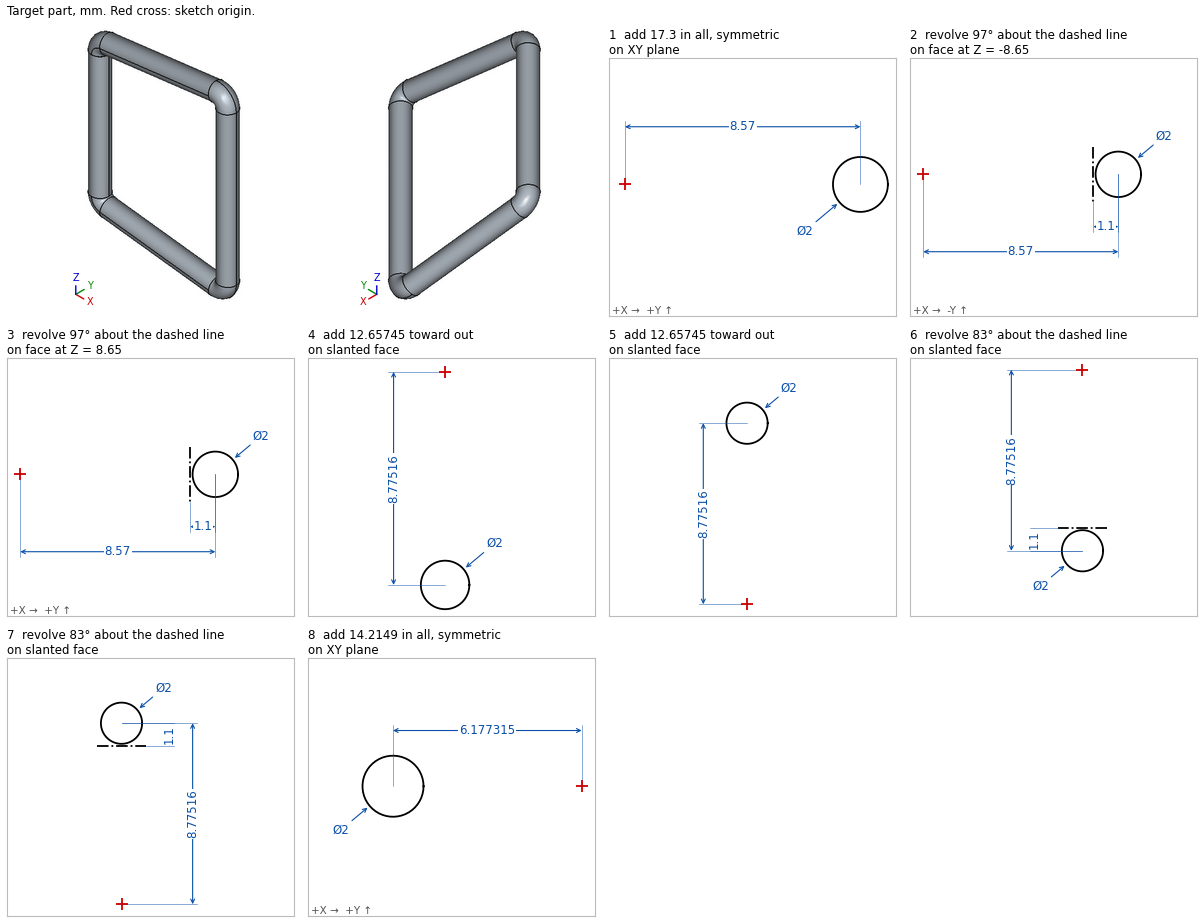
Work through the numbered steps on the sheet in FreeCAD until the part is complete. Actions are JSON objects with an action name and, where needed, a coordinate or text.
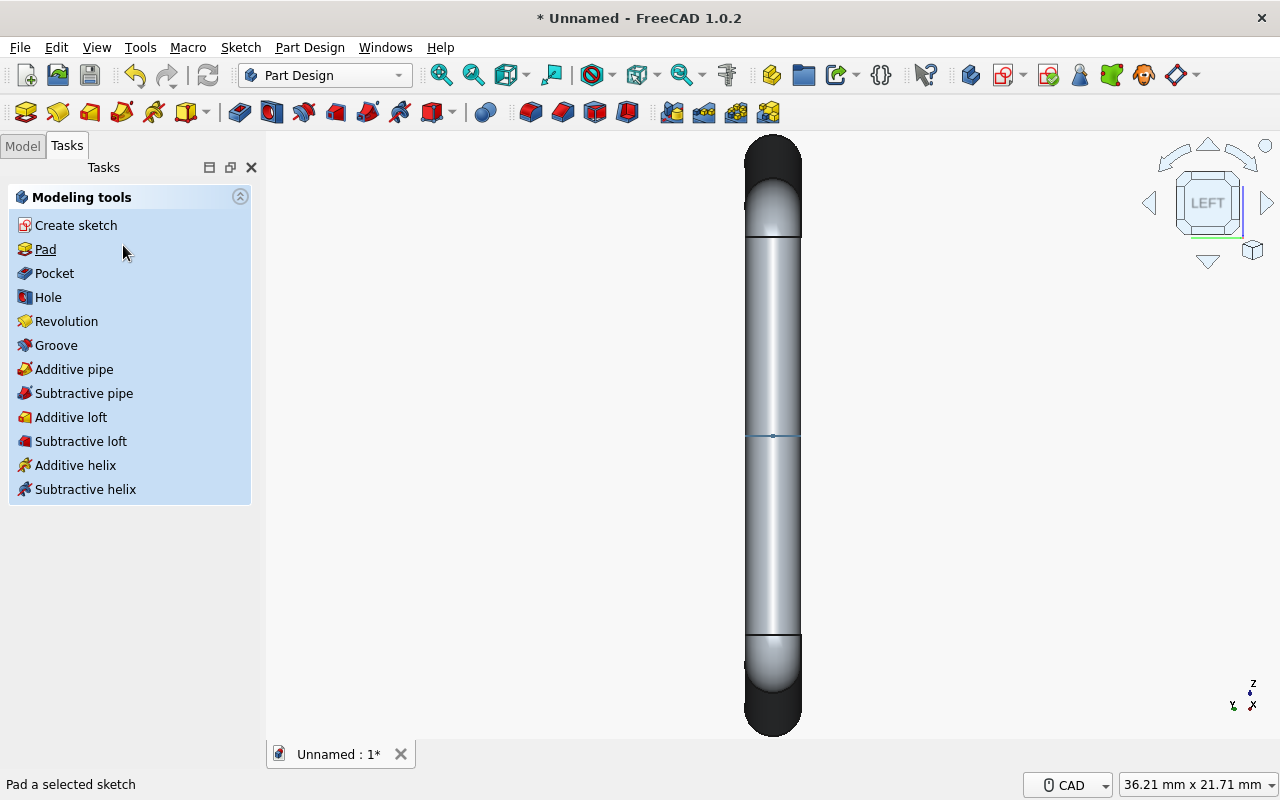
{"action": "left_click", "coordinate": [26, 112]}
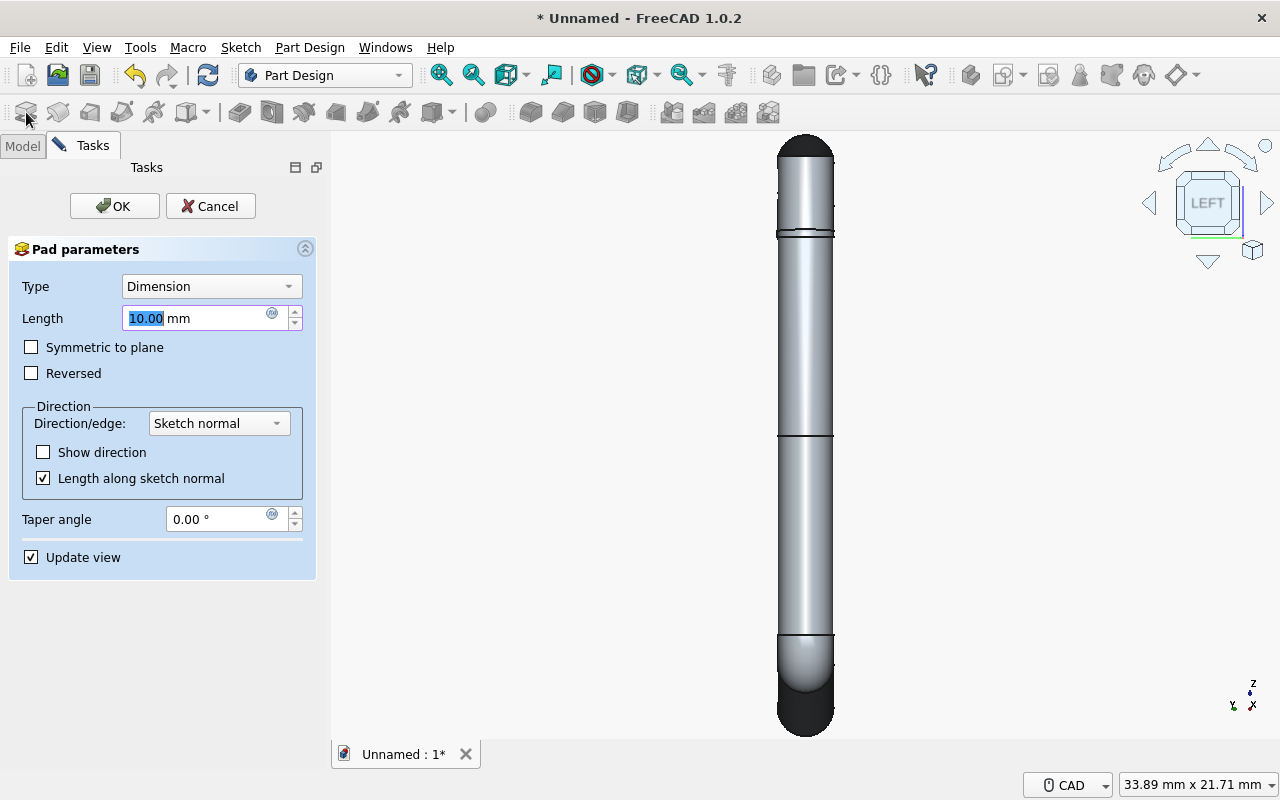
{"action": "type", "text": "14.2149"}
{"action": "key", "text": "Tab"}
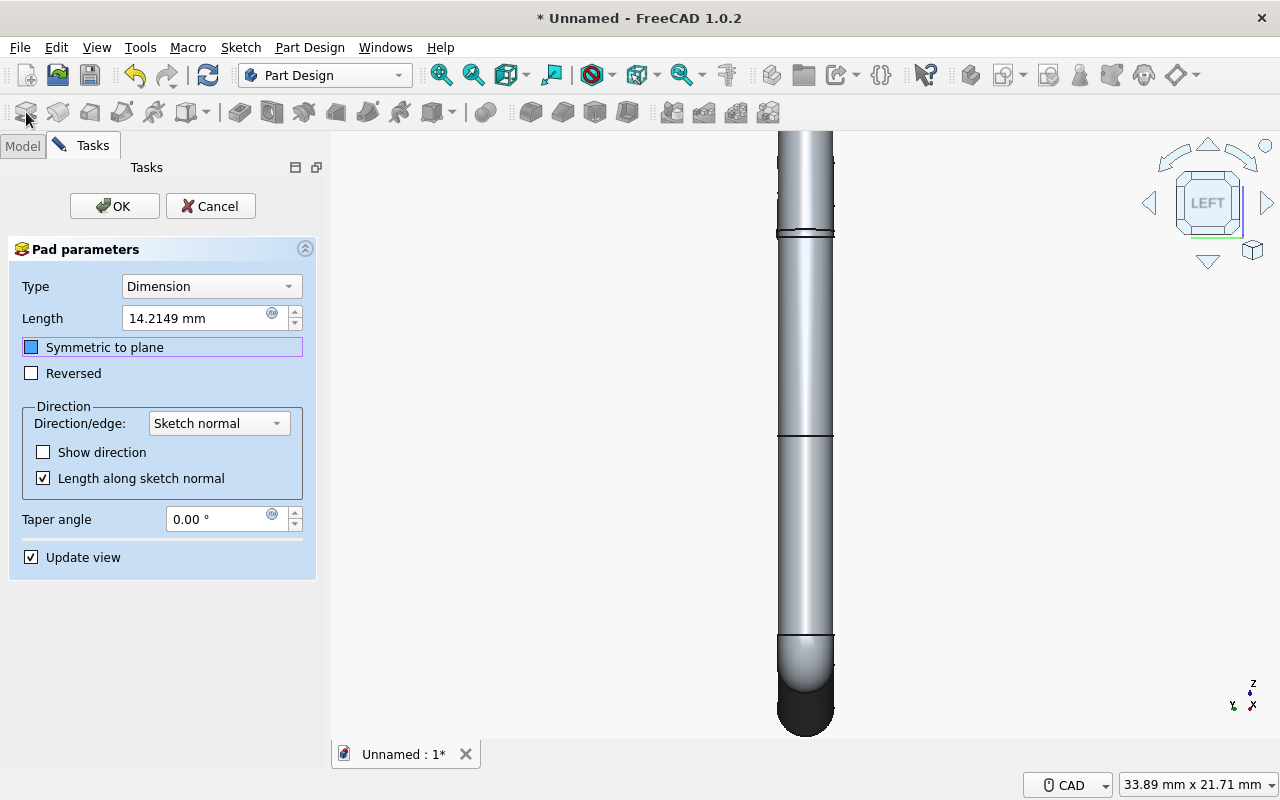
{"action": "left_click", "coordinate": [30, 347]}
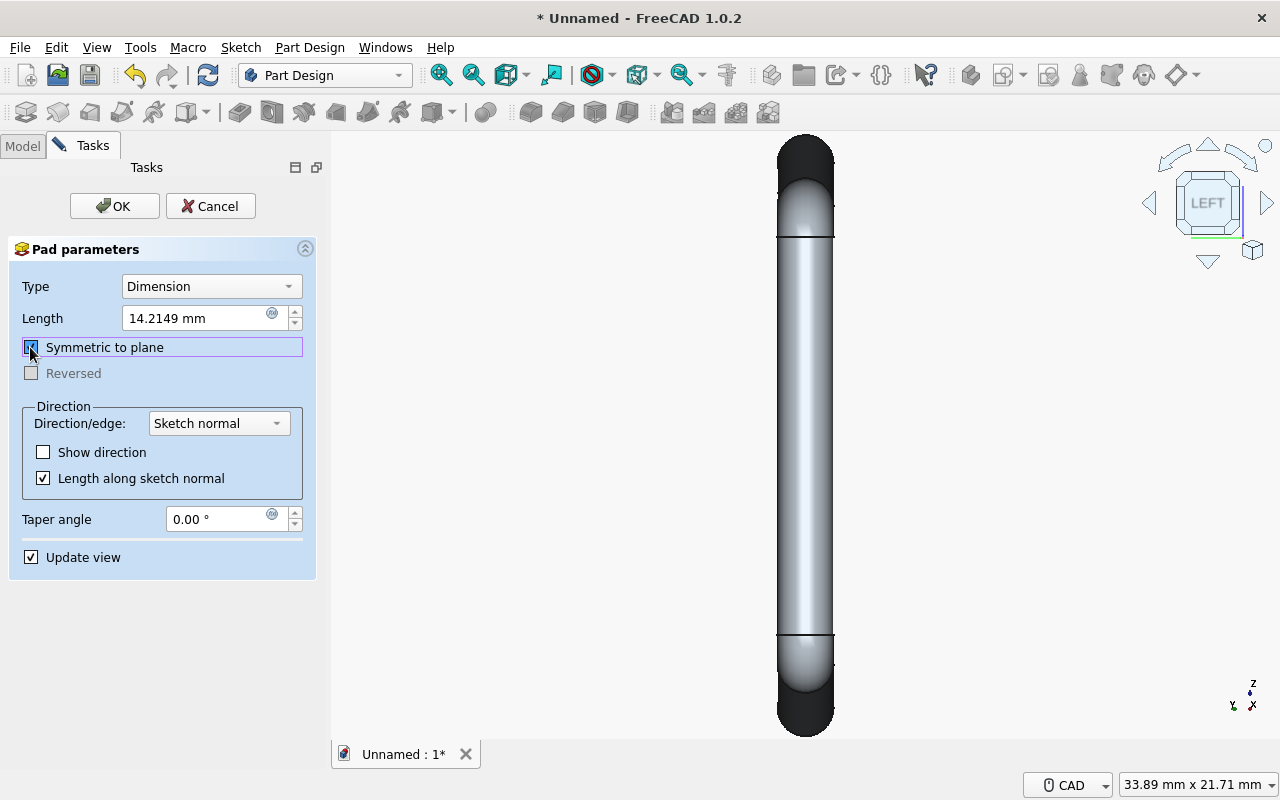
{"action": "left_click", "coordinate": [115, 206]}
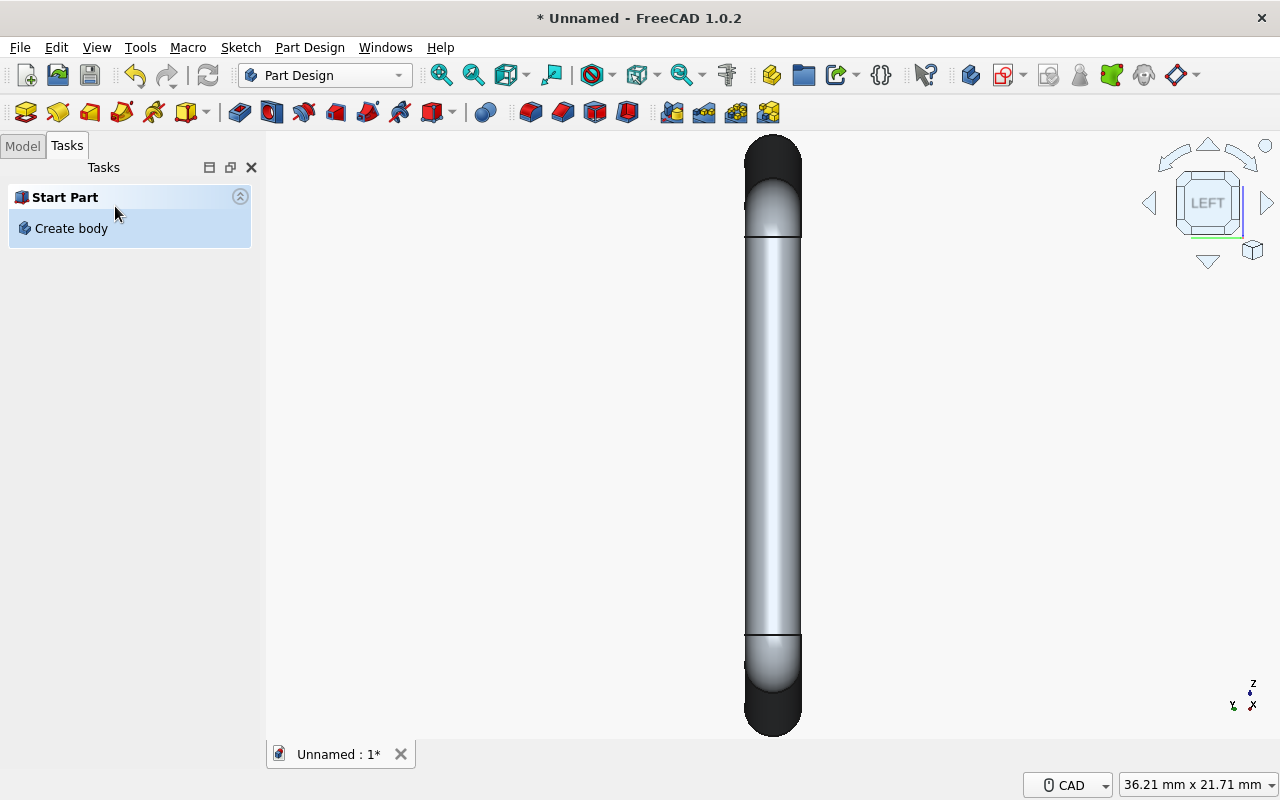
{"action": "key", "text": "0"}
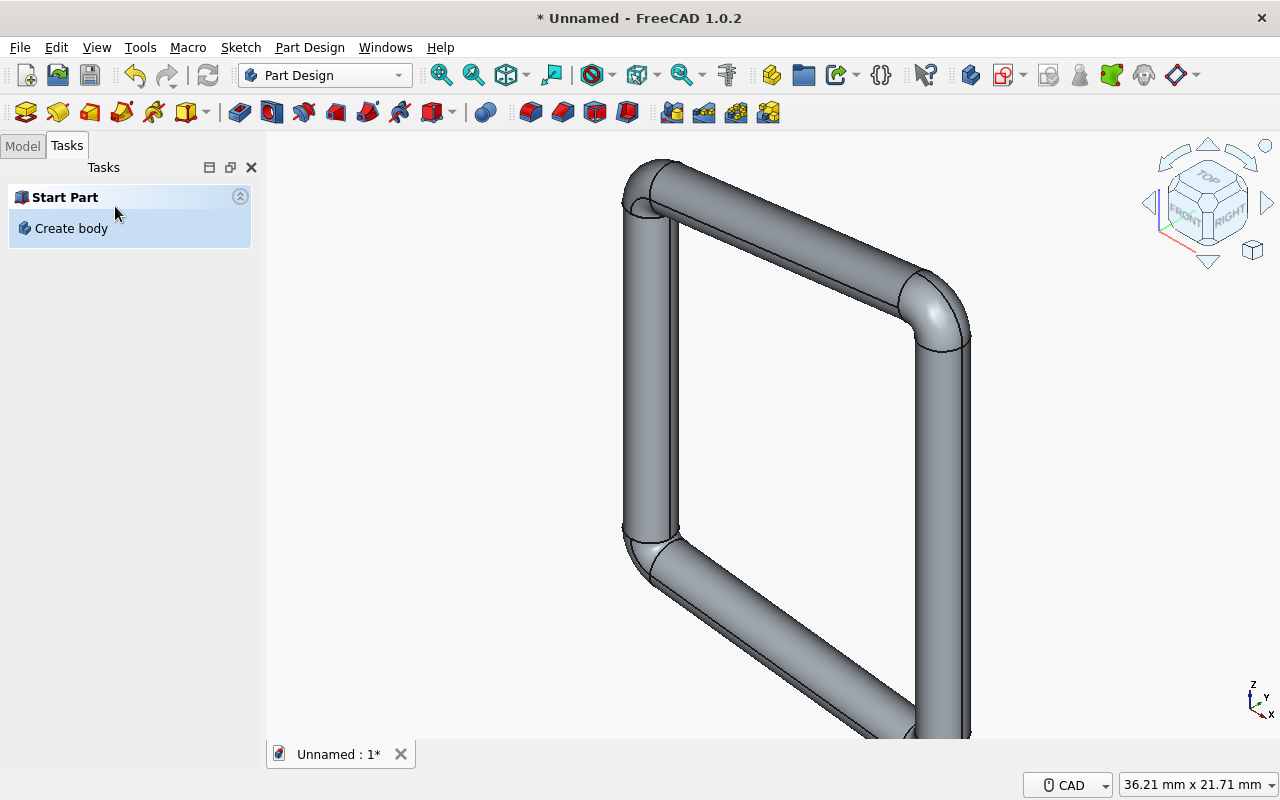
{"action": "left_click", "coordinate": [442, 76]}